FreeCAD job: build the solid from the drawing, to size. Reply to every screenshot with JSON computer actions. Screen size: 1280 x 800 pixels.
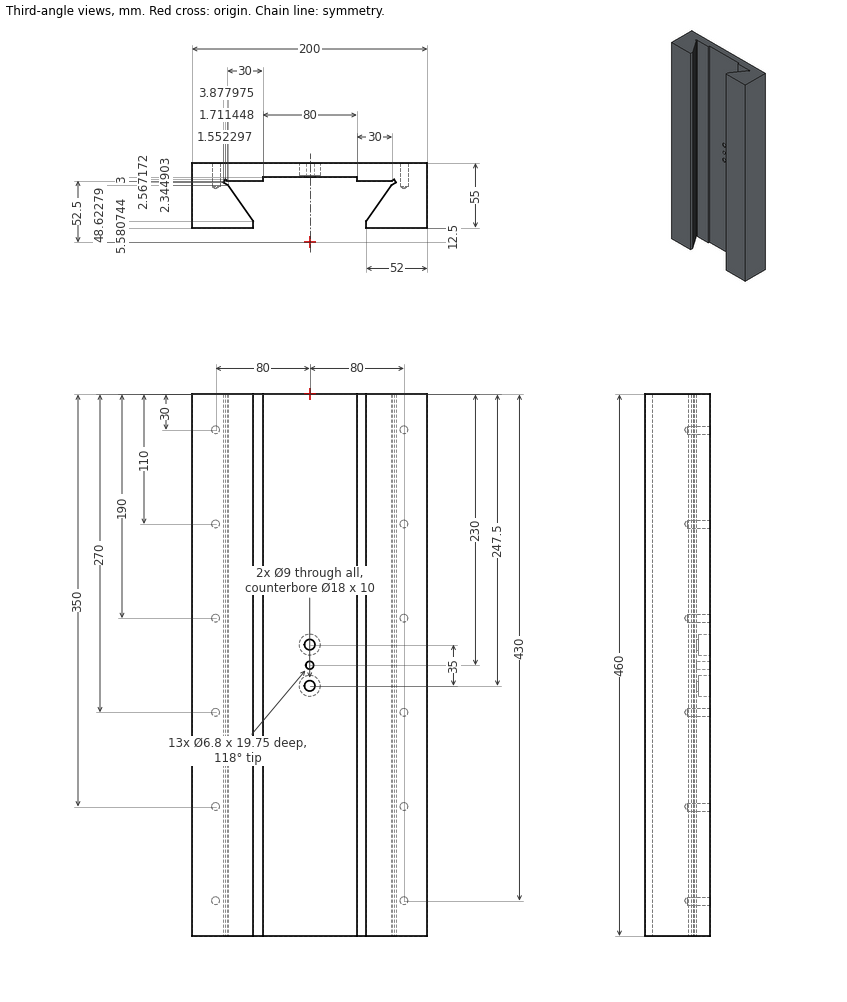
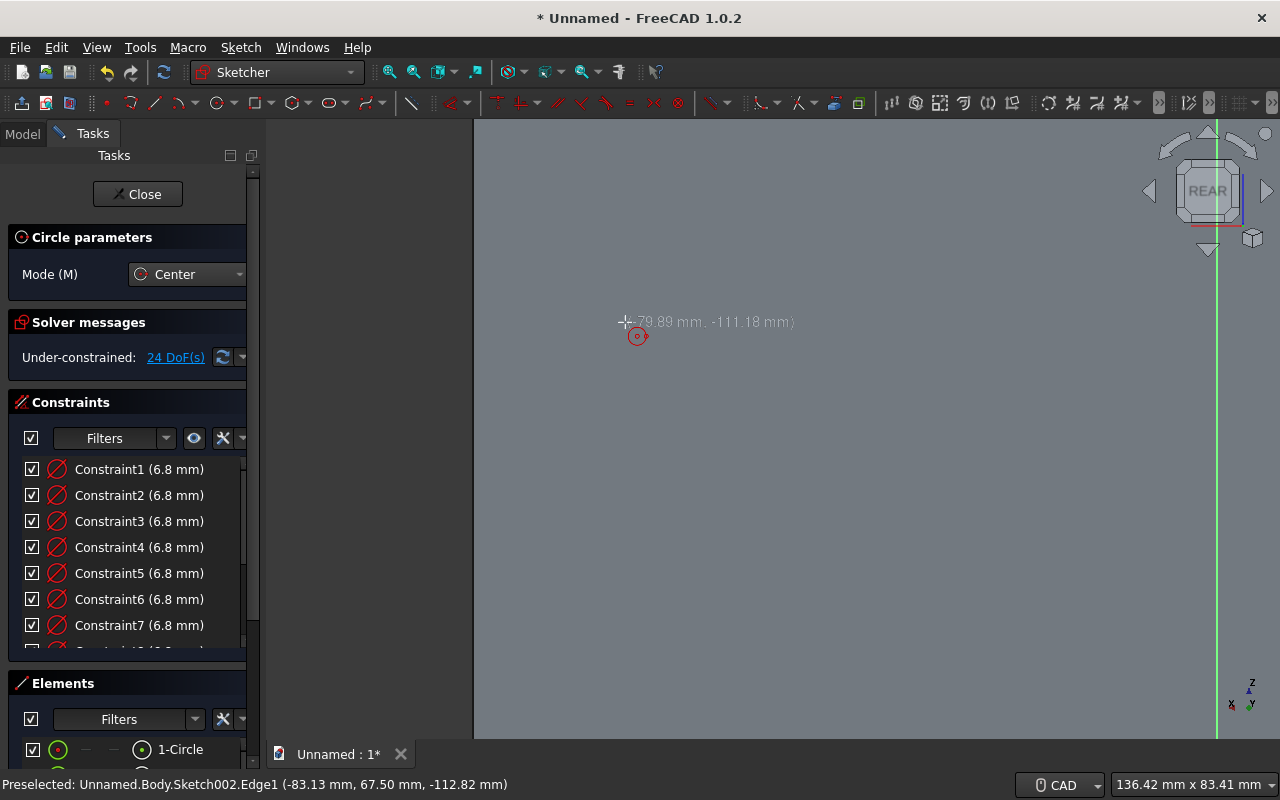
{"action": "scroll", "coordinate": [624, 322], "scroll_direction": "down", "scroll_amount": 10}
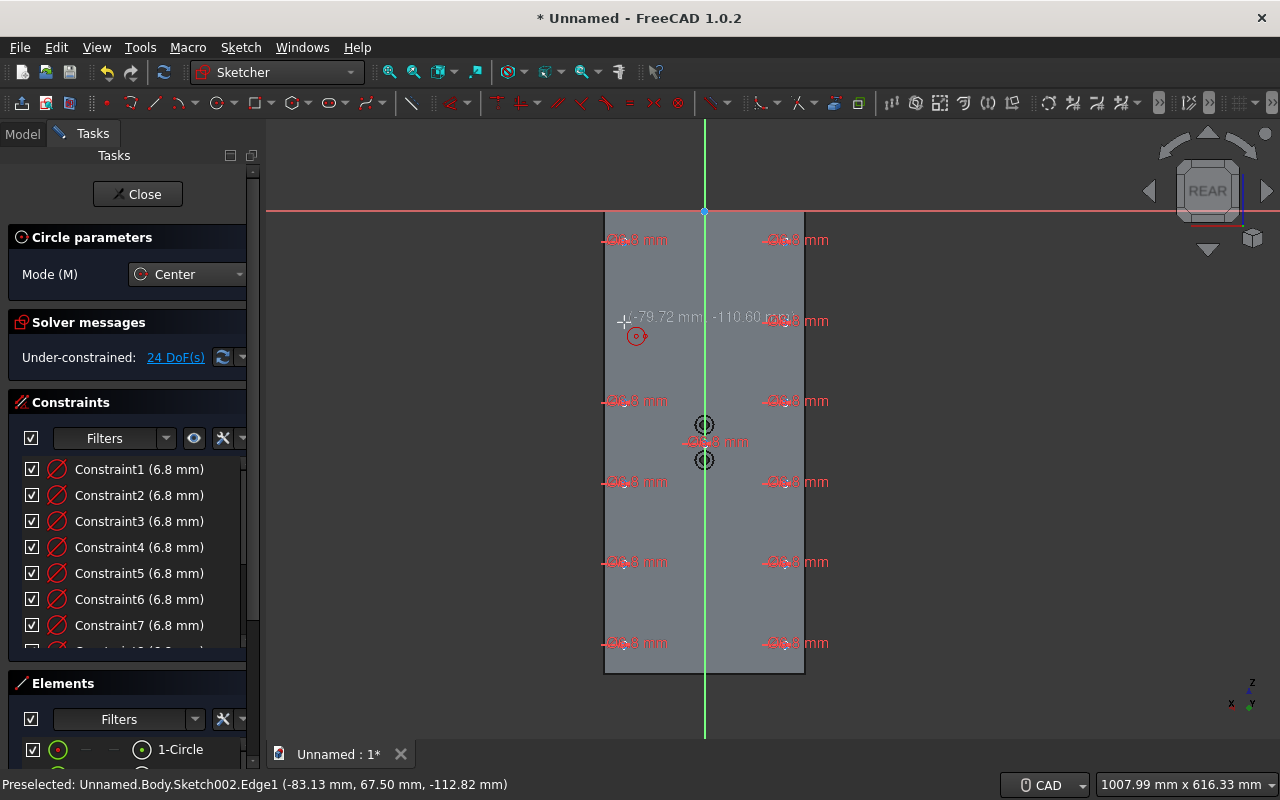
{"action": "left_click", "coordinate": [624, 322]}
{"action": "mouse_move", "coordinate": [626, 319]}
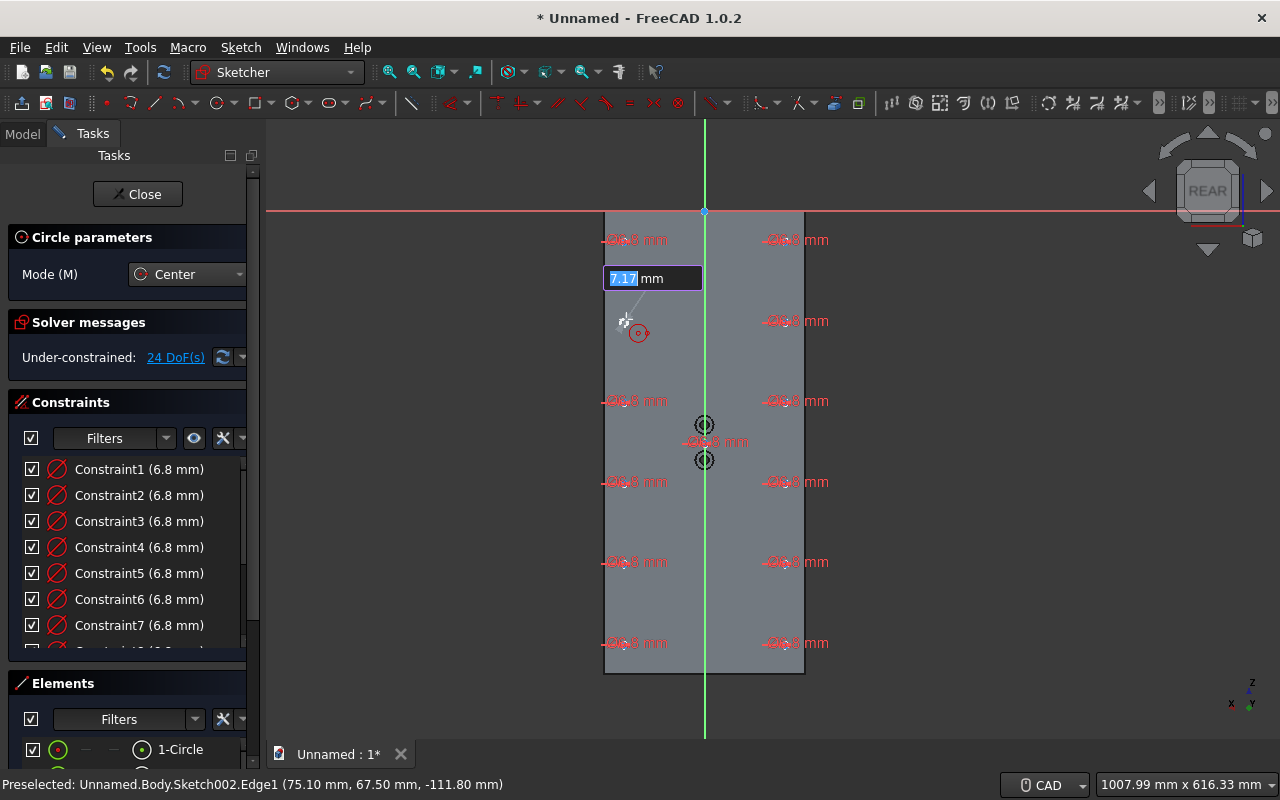
{"action": "type", "text": "6.8"}
{"action": "key", "text": "Return"}
{"action": "key", "text": "Escape"}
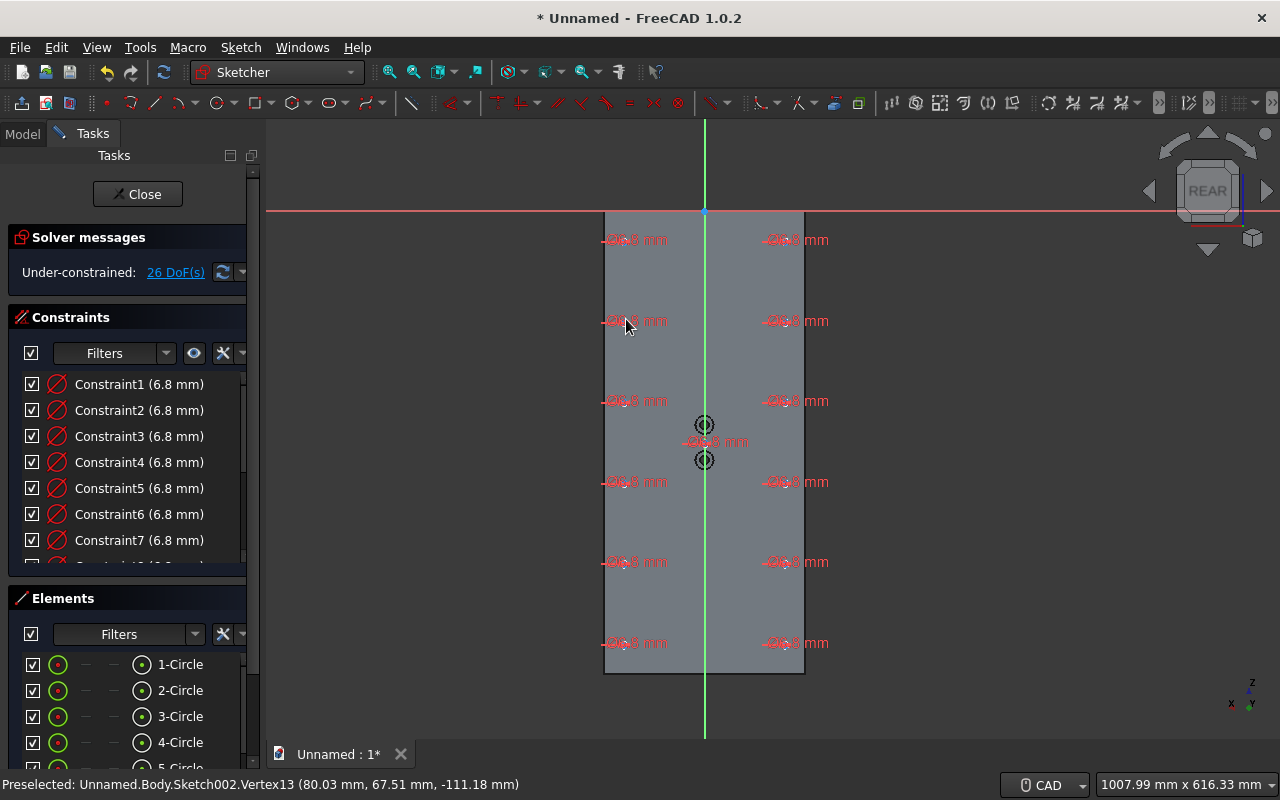
{"action": "left_click", "coordinate": [705, 444]}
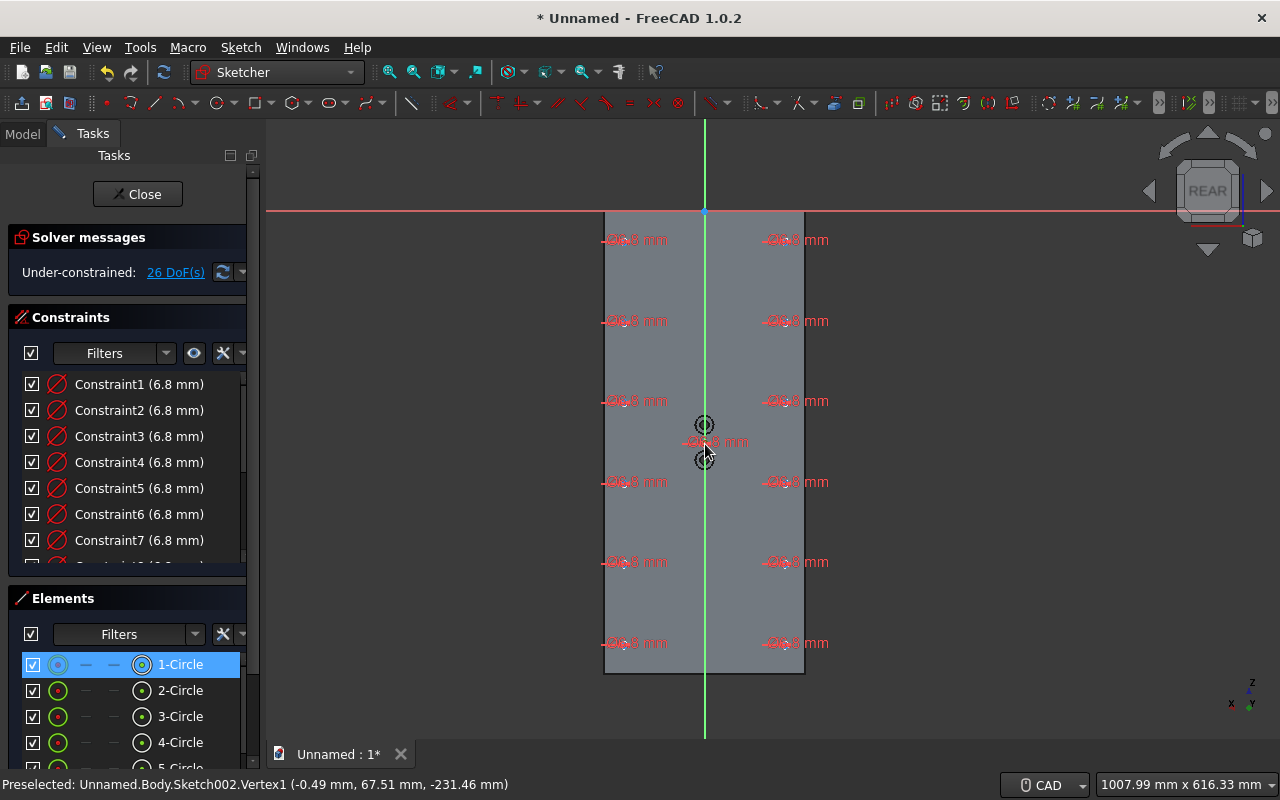
{"action": "left_click", "coordinate": [705, 671]}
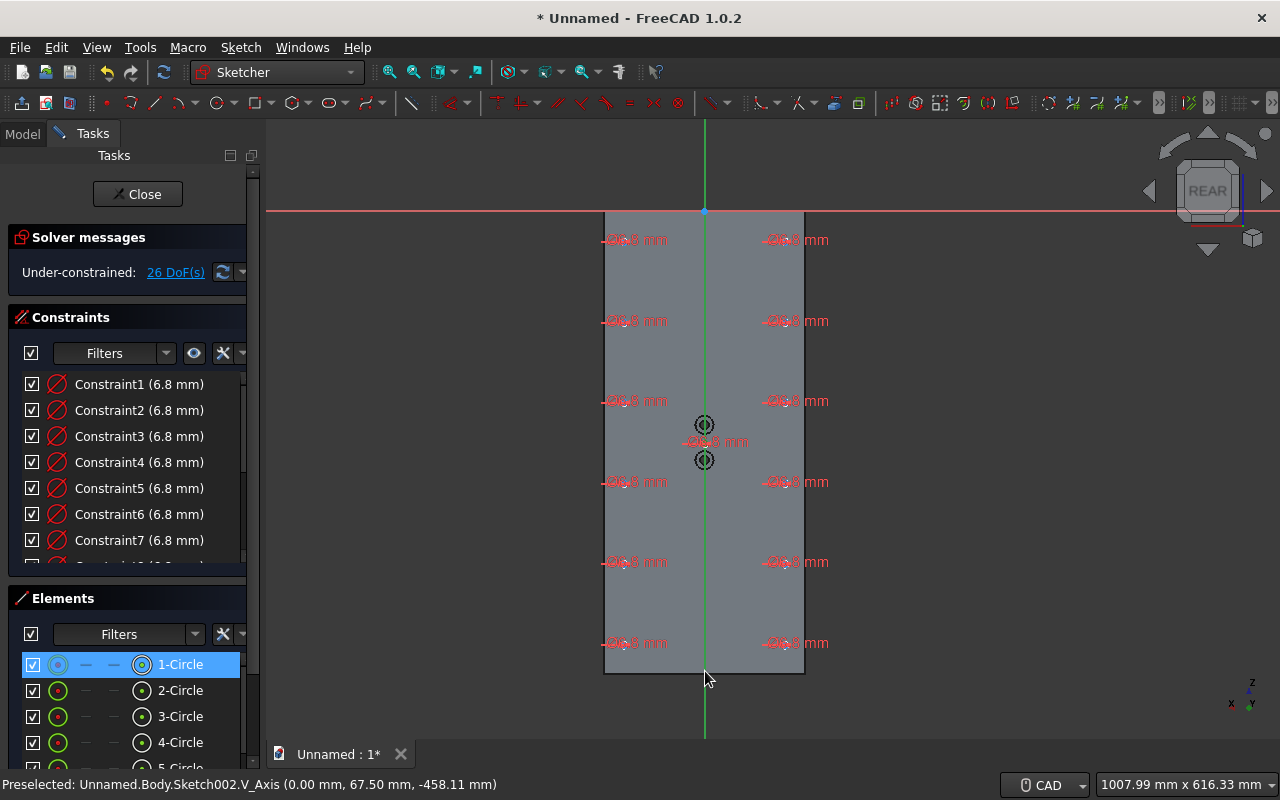
{"action": "left_click", "coordinate": [498, 104]}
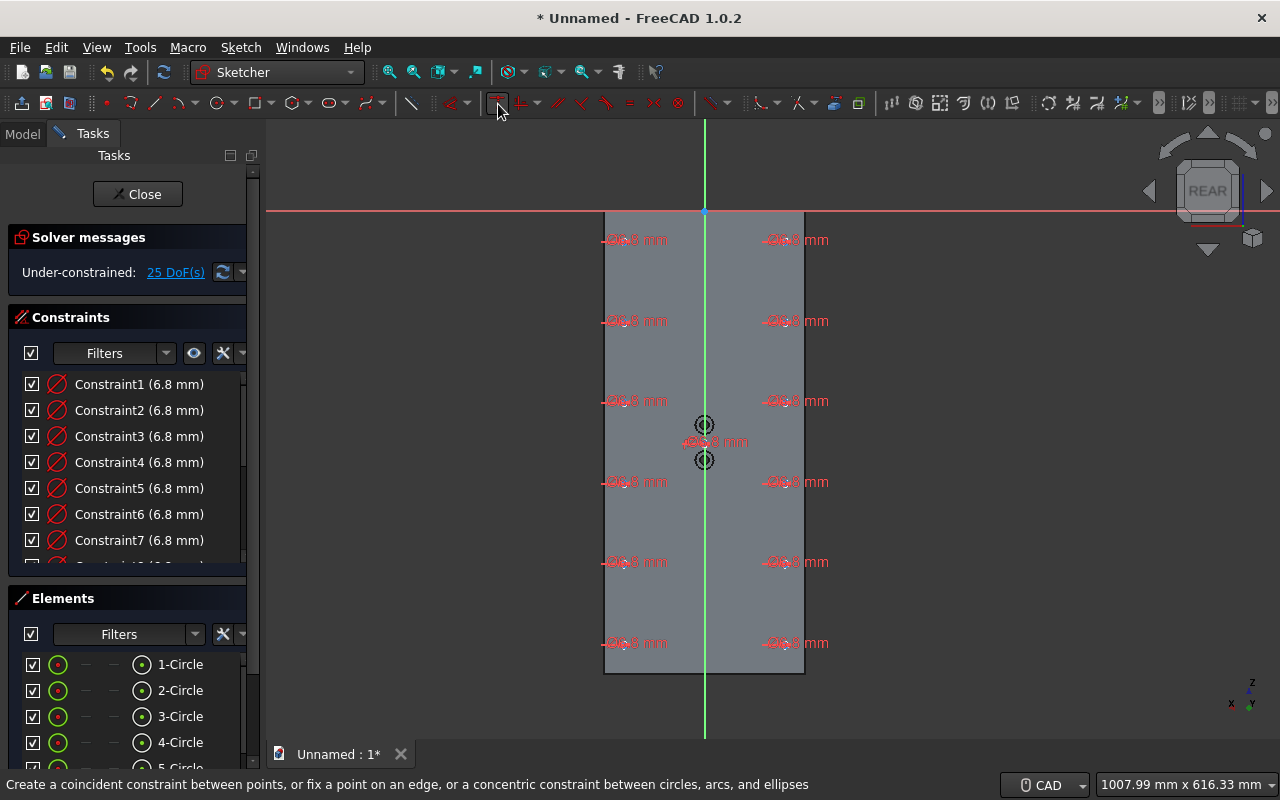
{"action": "left_click", "coordinate": [785, 242]}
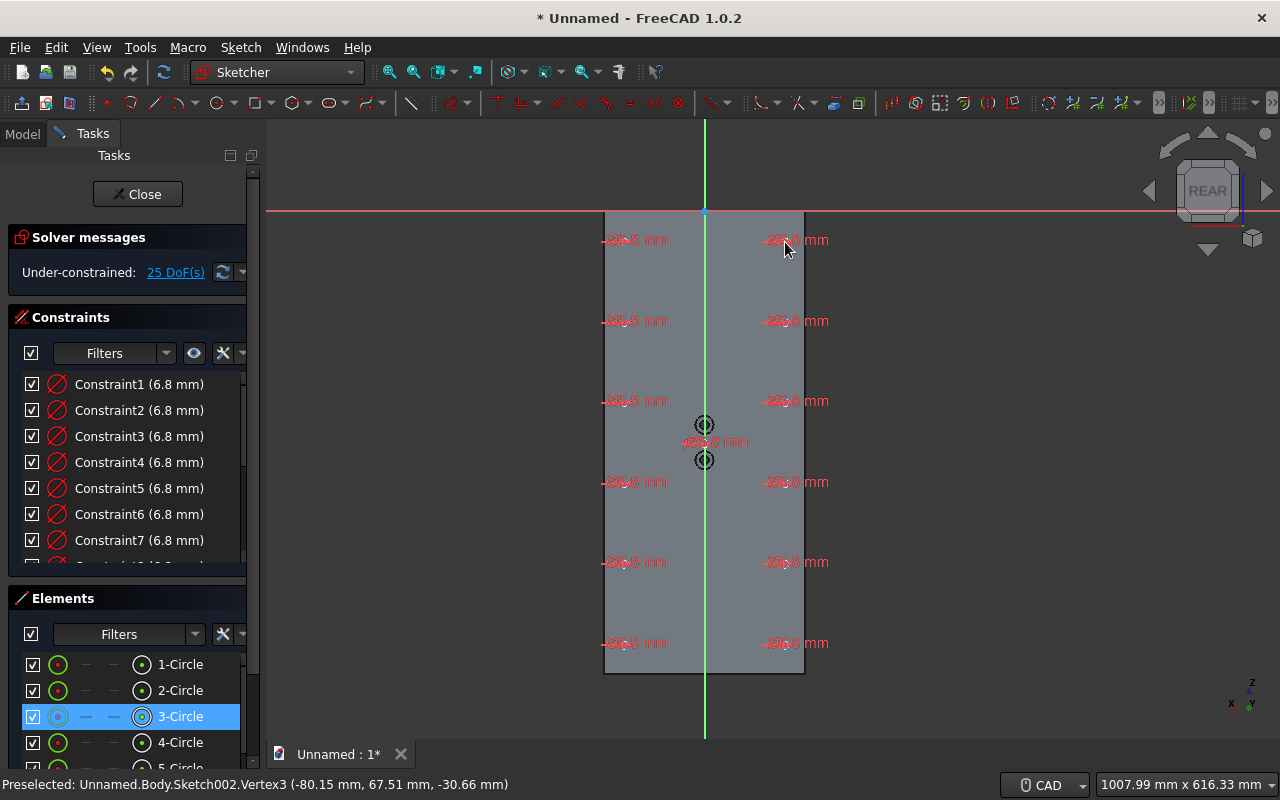
{"action": "left_click", "coordinate": [785, 645]}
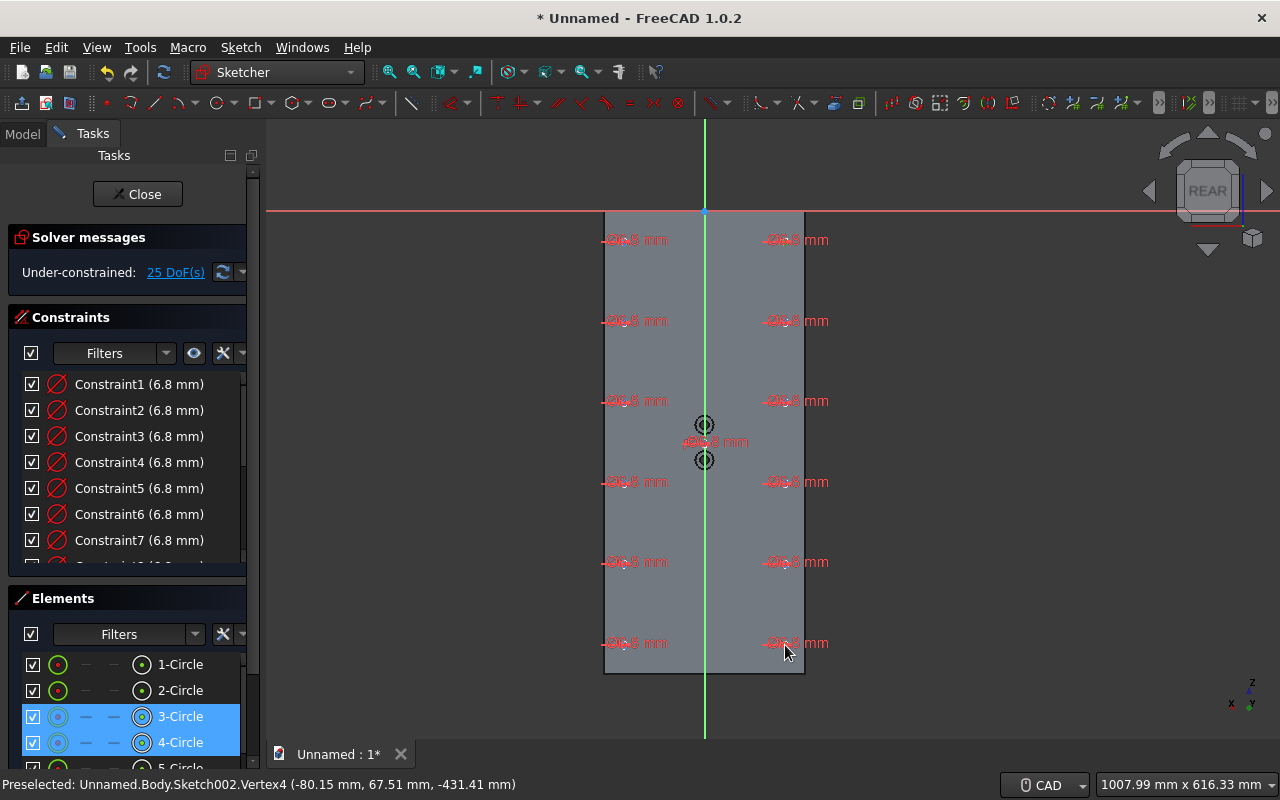
{"action": "left_click", "coordinate": [540, 104]}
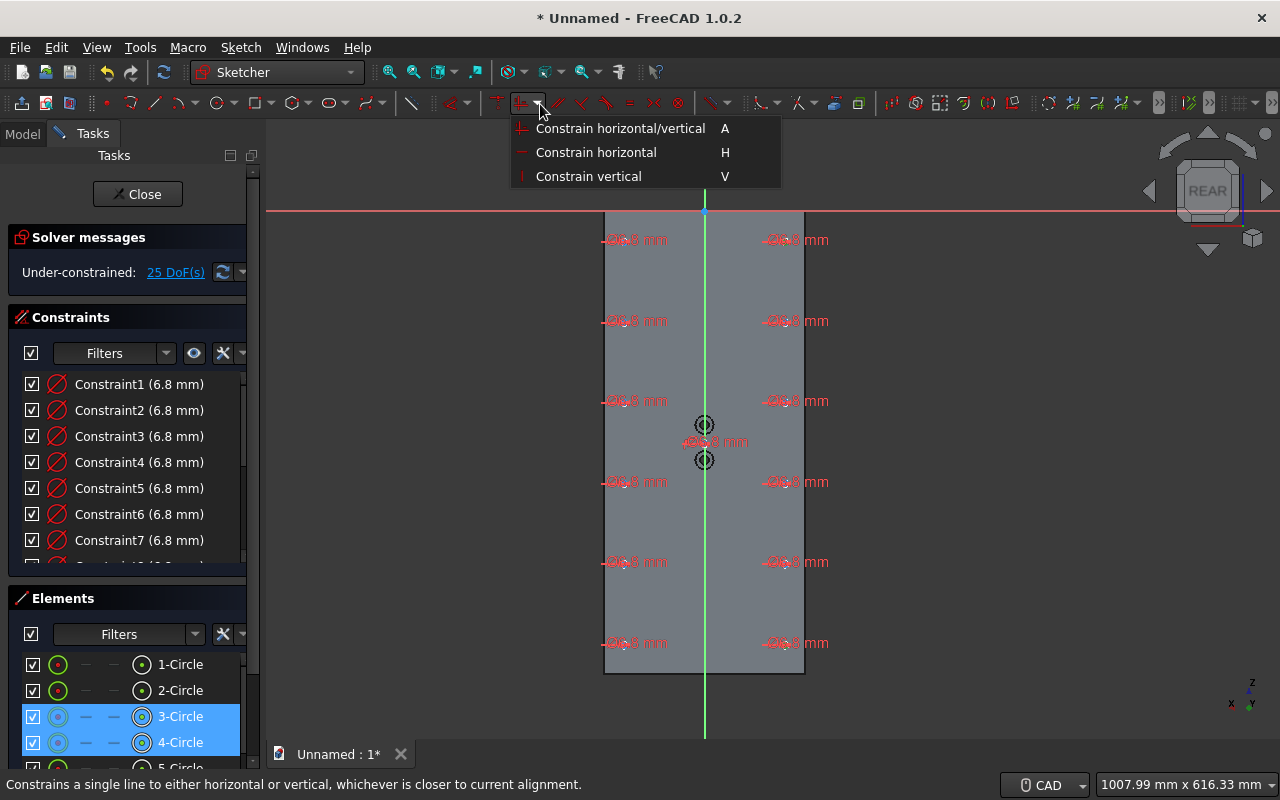
{"action": "left_click", "coordinate": [646, 176]}